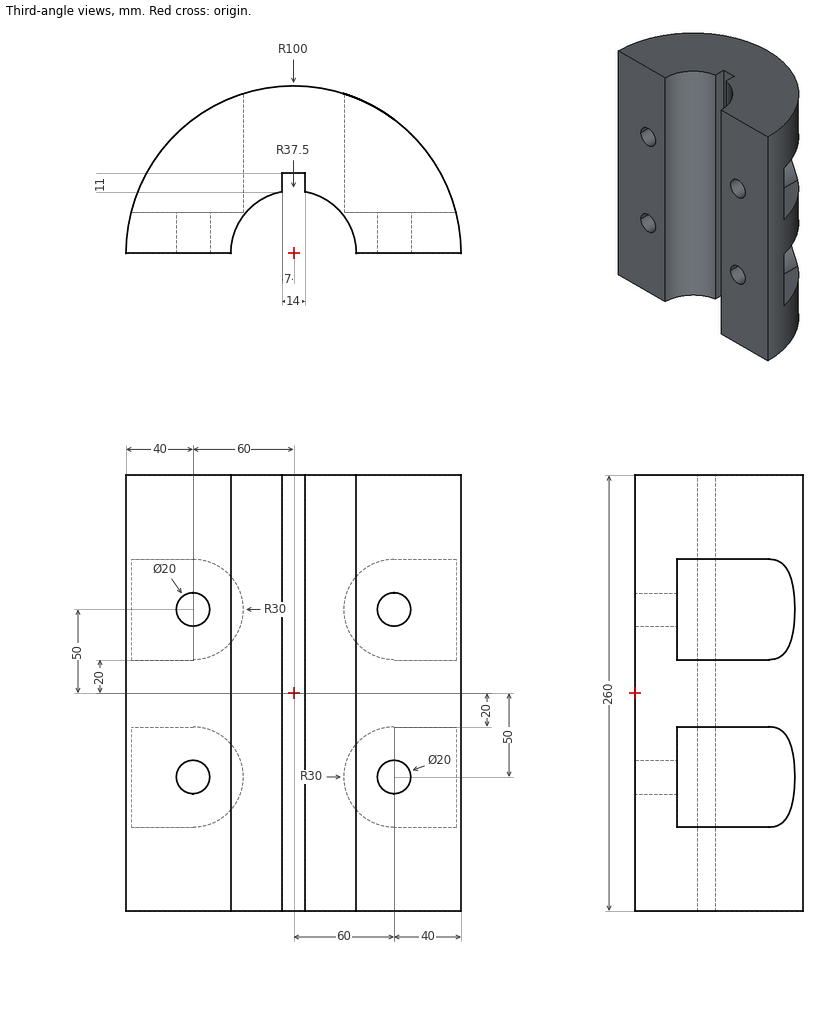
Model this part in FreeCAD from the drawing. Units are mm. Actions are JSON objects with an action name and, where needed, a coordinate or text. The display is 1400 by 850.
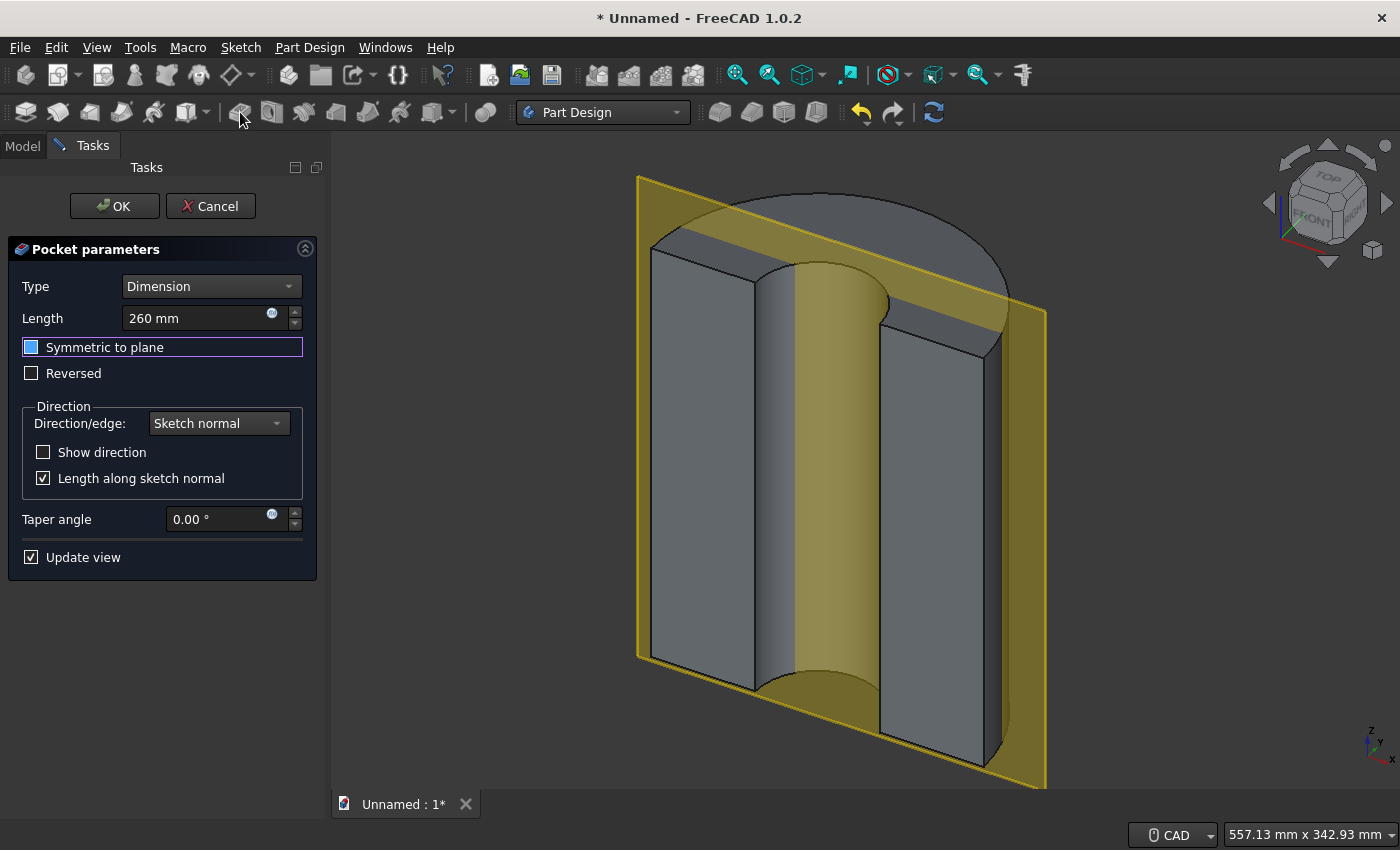
{"action": "left_click", "coordinate": [115, 206]}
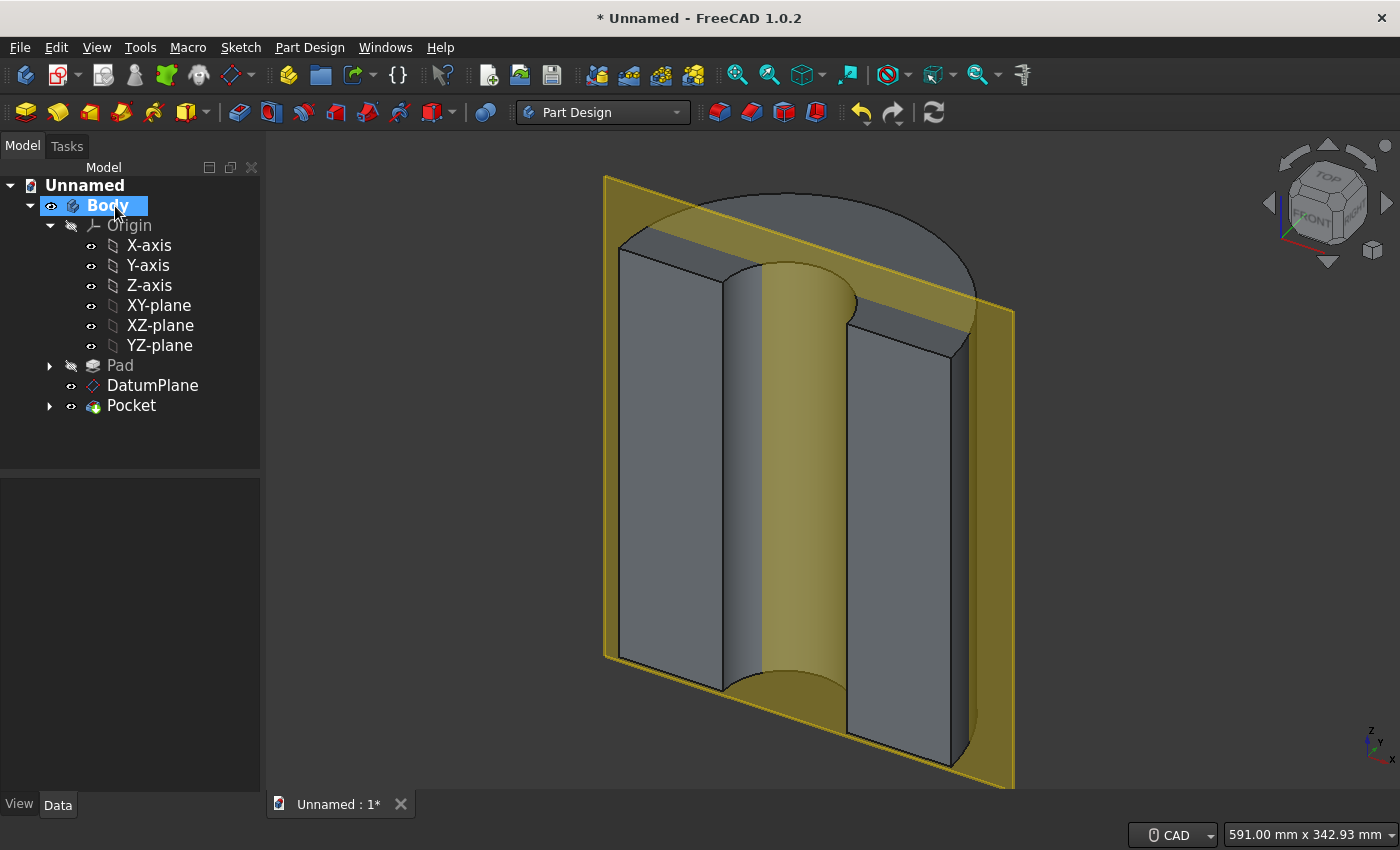
{"action": "left_click", "coordinate": [116, 386]}
{"action": "key", "text": "space"}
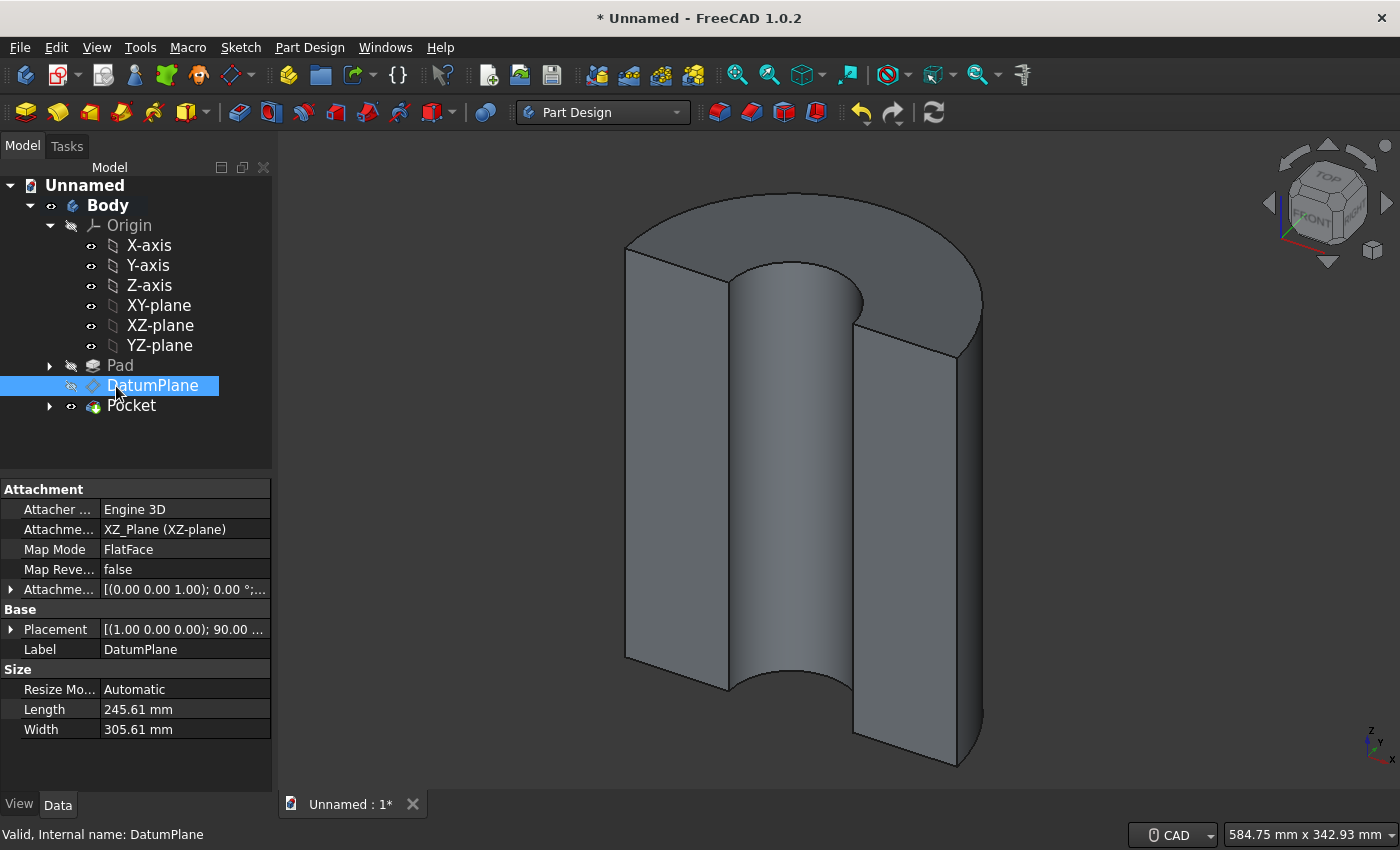
{"action": "left_click", "coordinate": [116, 406]}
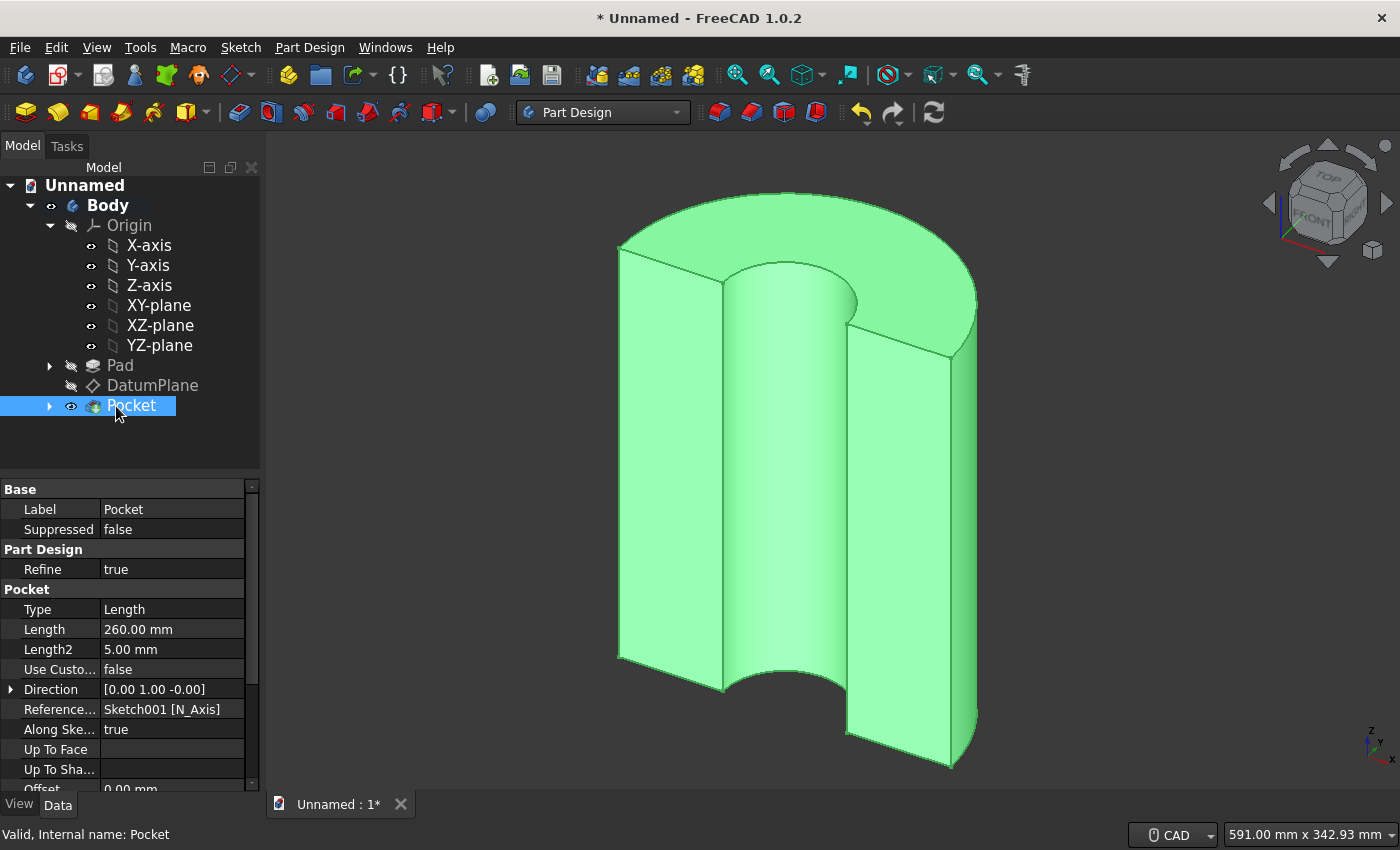
{"action": "left_click", "coordinate": [598, 76]}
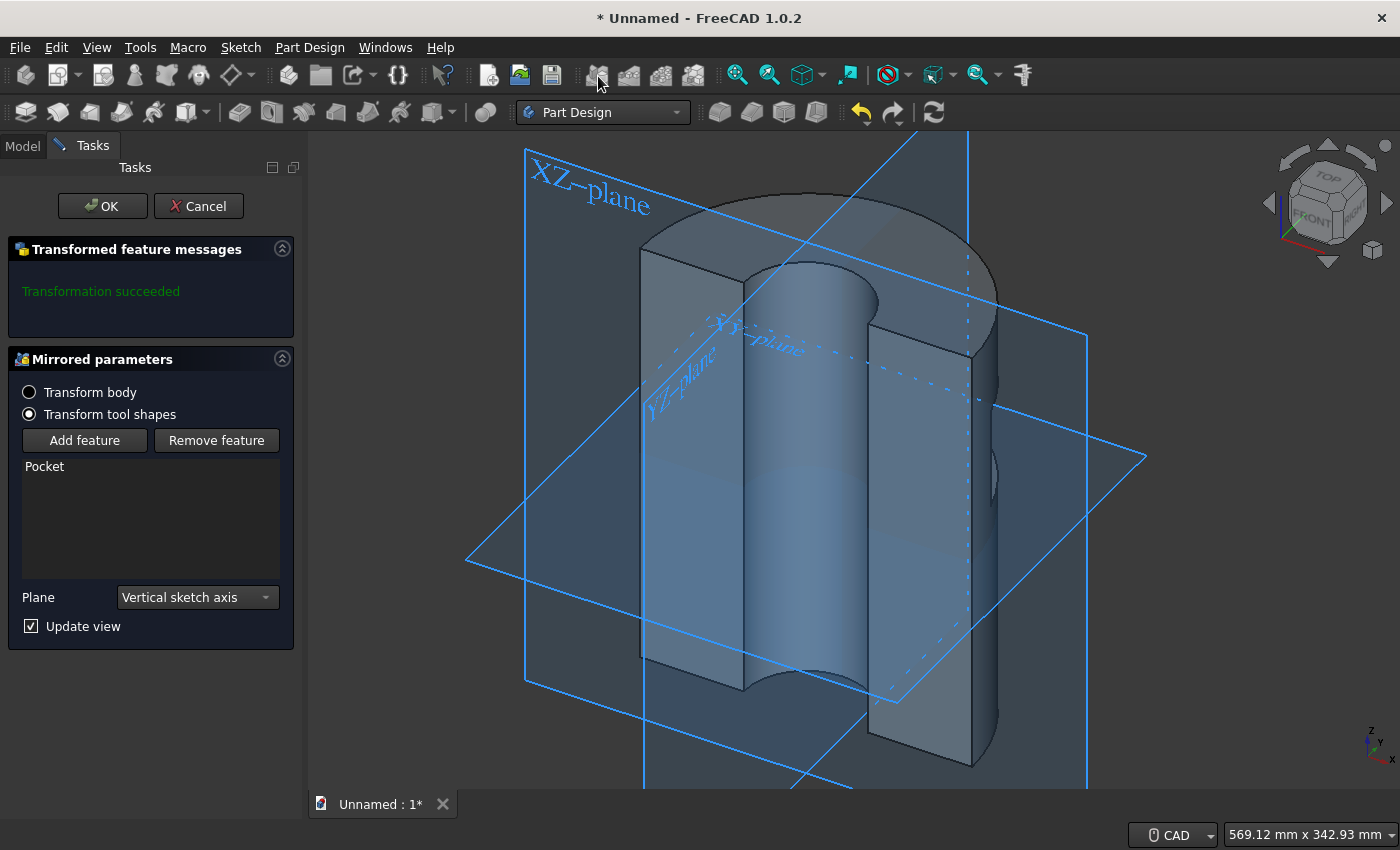
{"action": "left_click", "coordinate": [198, 598]}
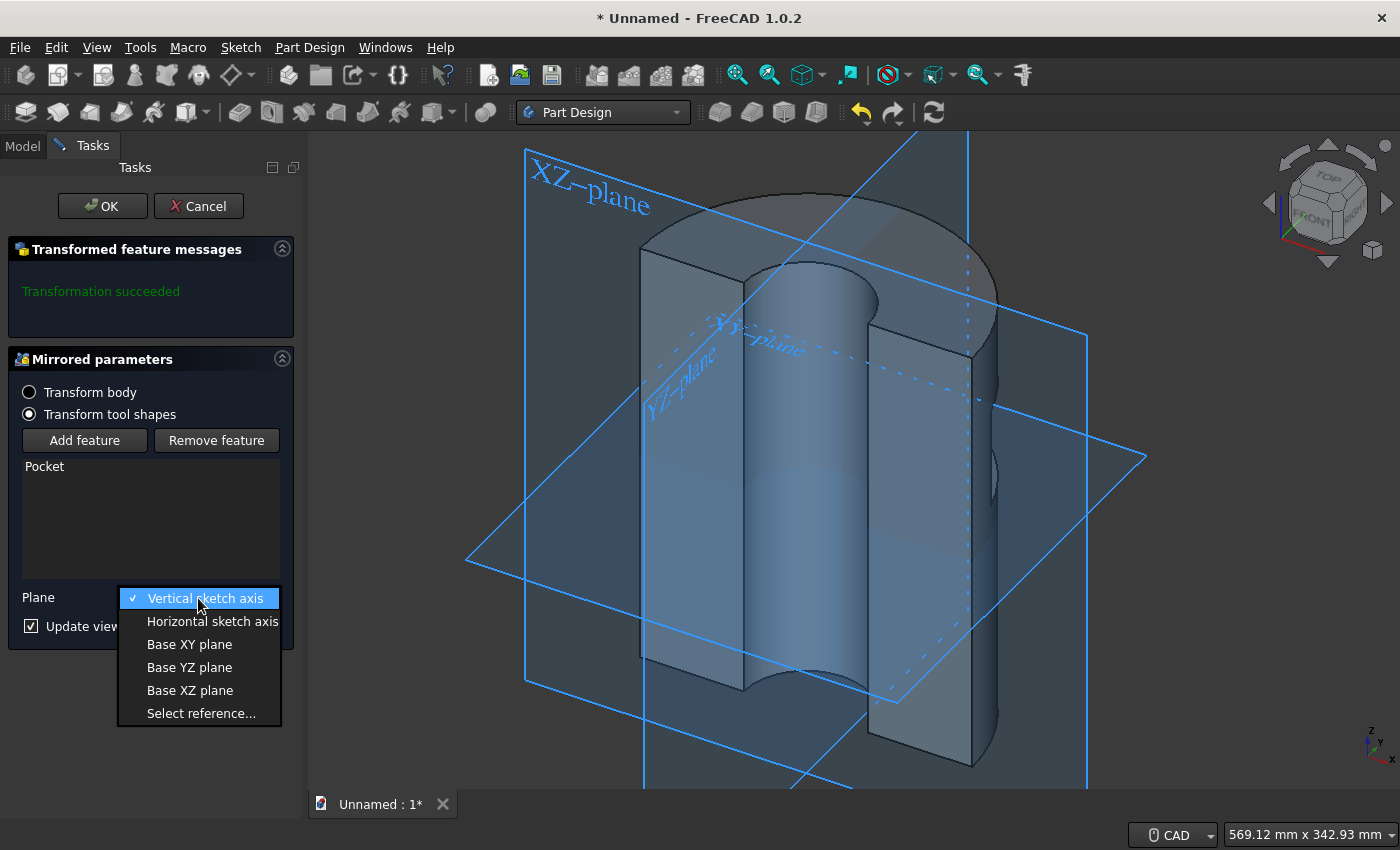
{"action": "left_click", "coordinate": [198, 644]}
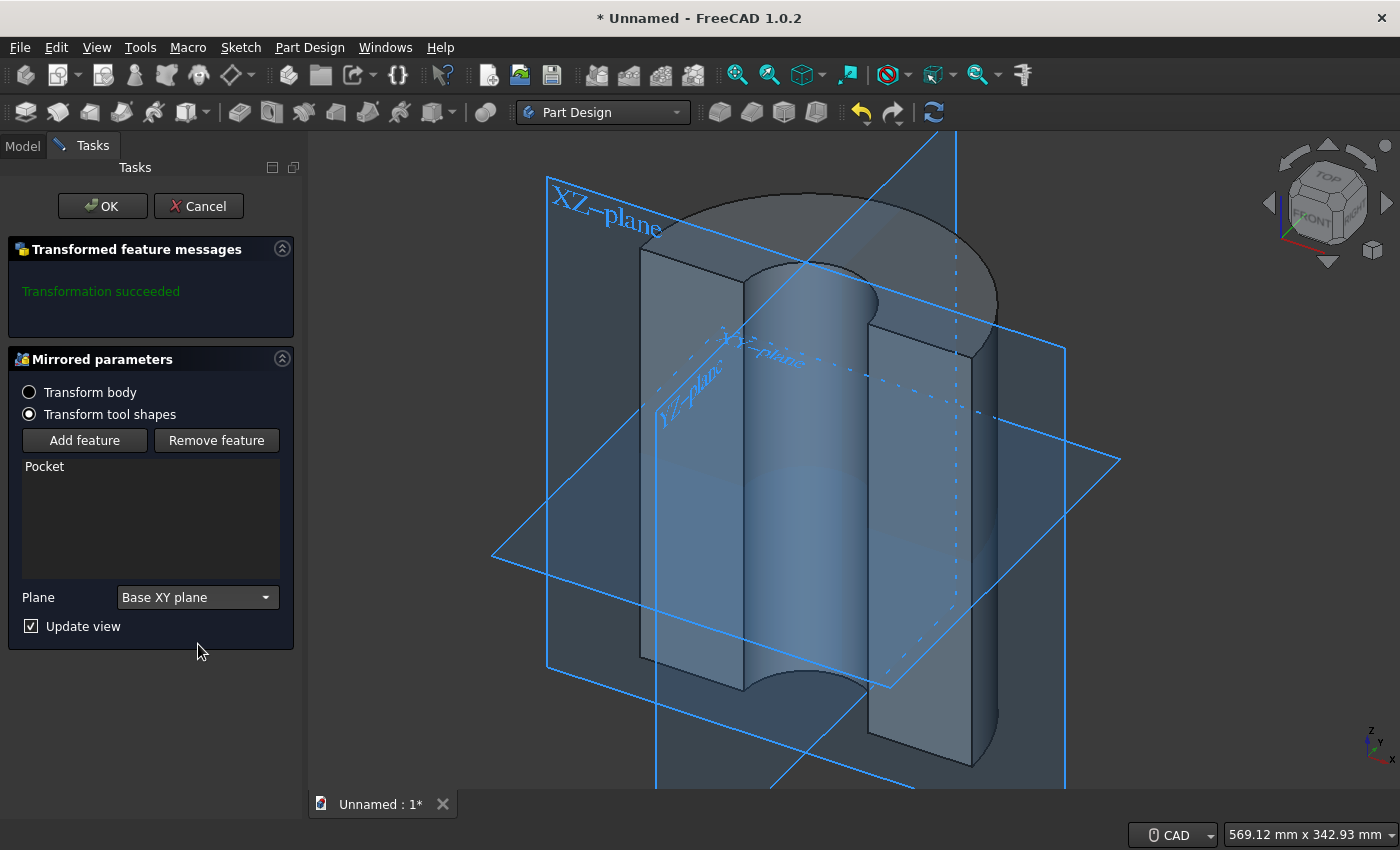
{"action": "left_click", "coordinate": [103, 206]}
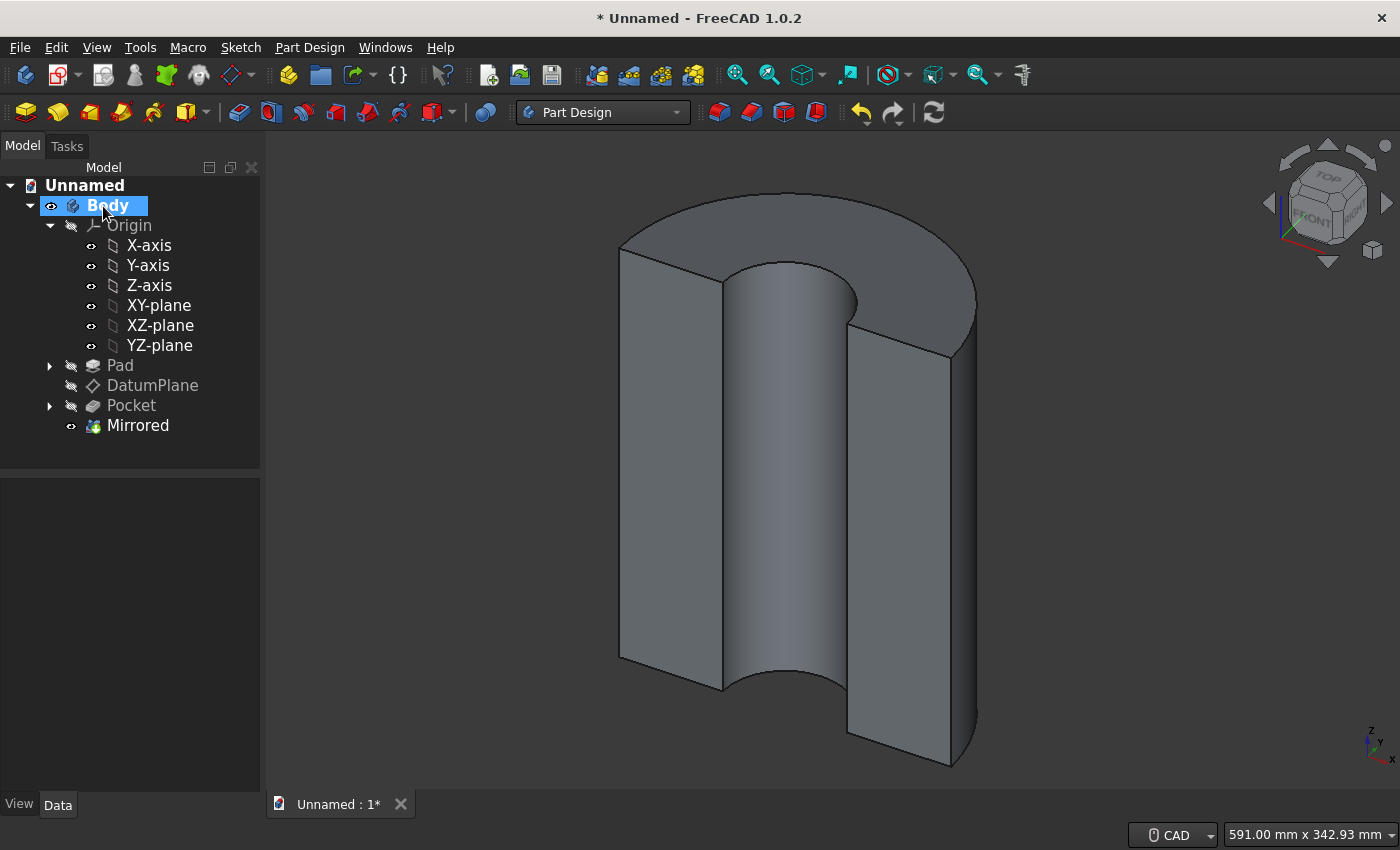
{"action": "left_click", "coordinate": [116, 406]}